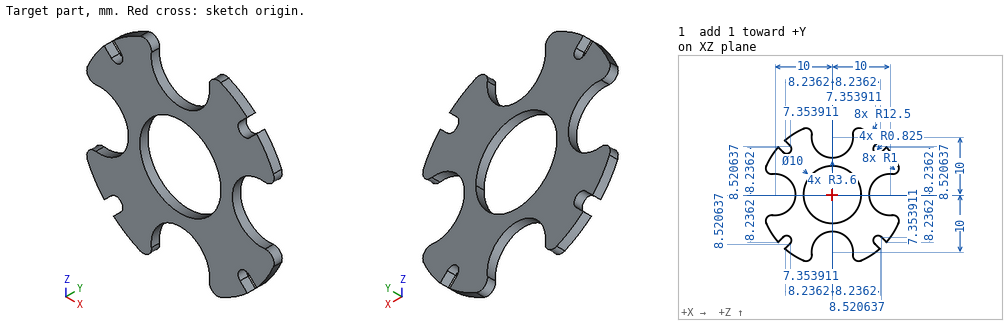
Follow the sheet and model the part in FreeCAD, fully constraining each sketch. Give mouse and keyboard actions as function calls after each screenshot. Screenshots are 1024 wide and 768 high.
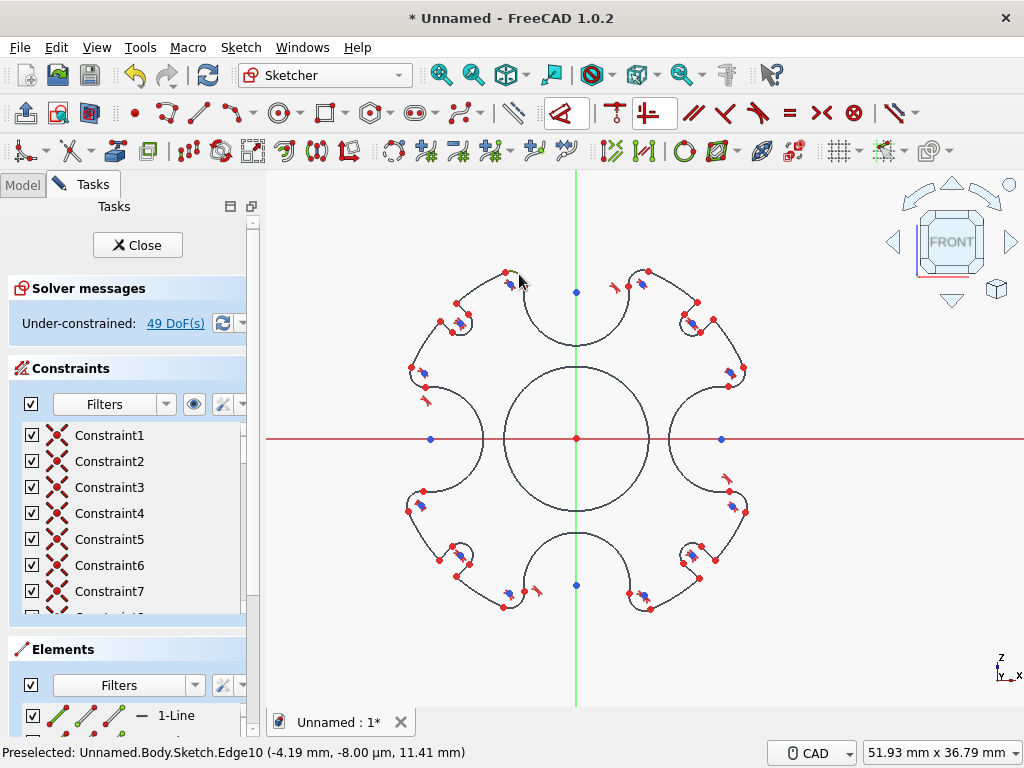
click(634, 273)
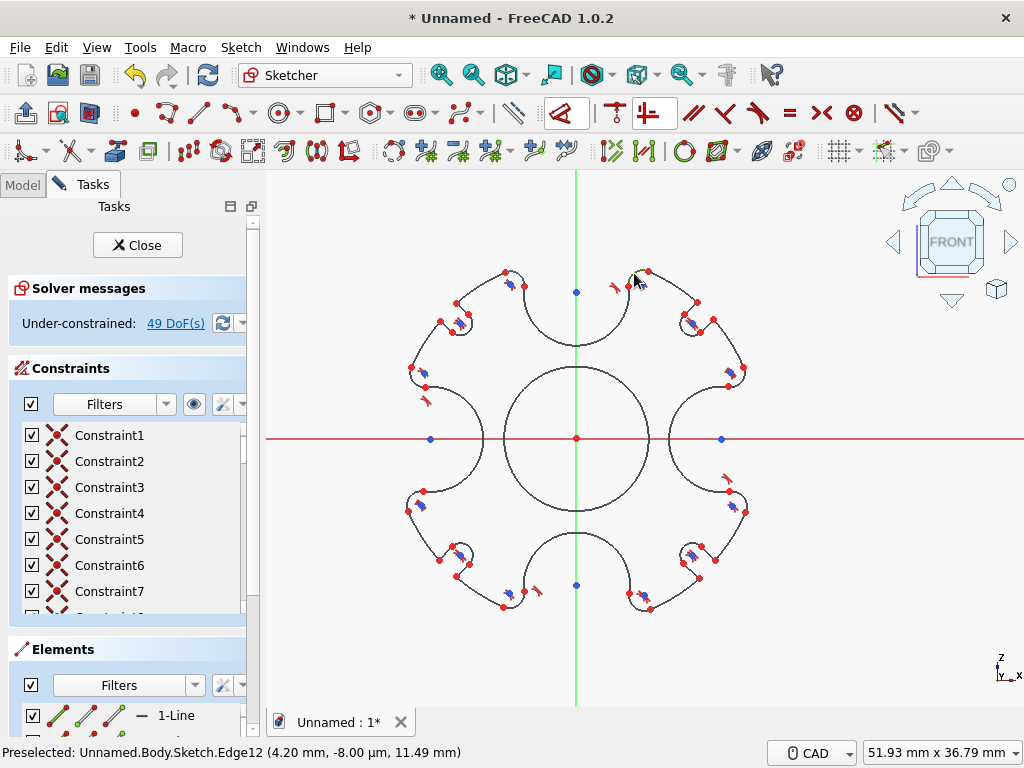
click(742, 381)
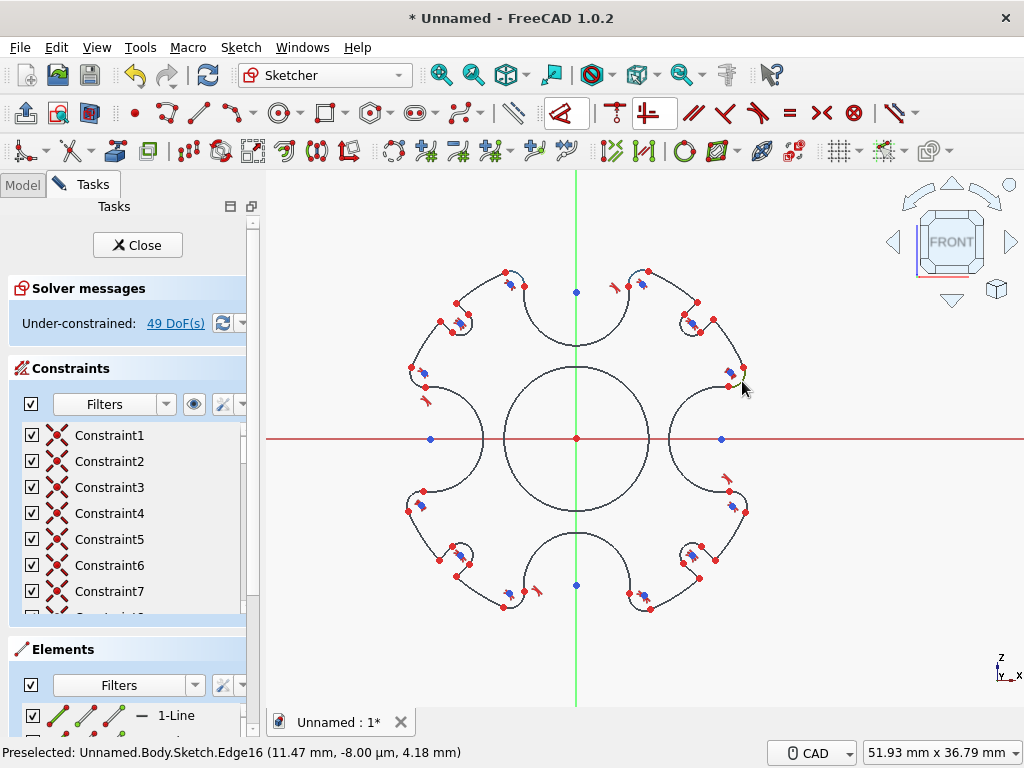
scroll(747, 503, up, 2)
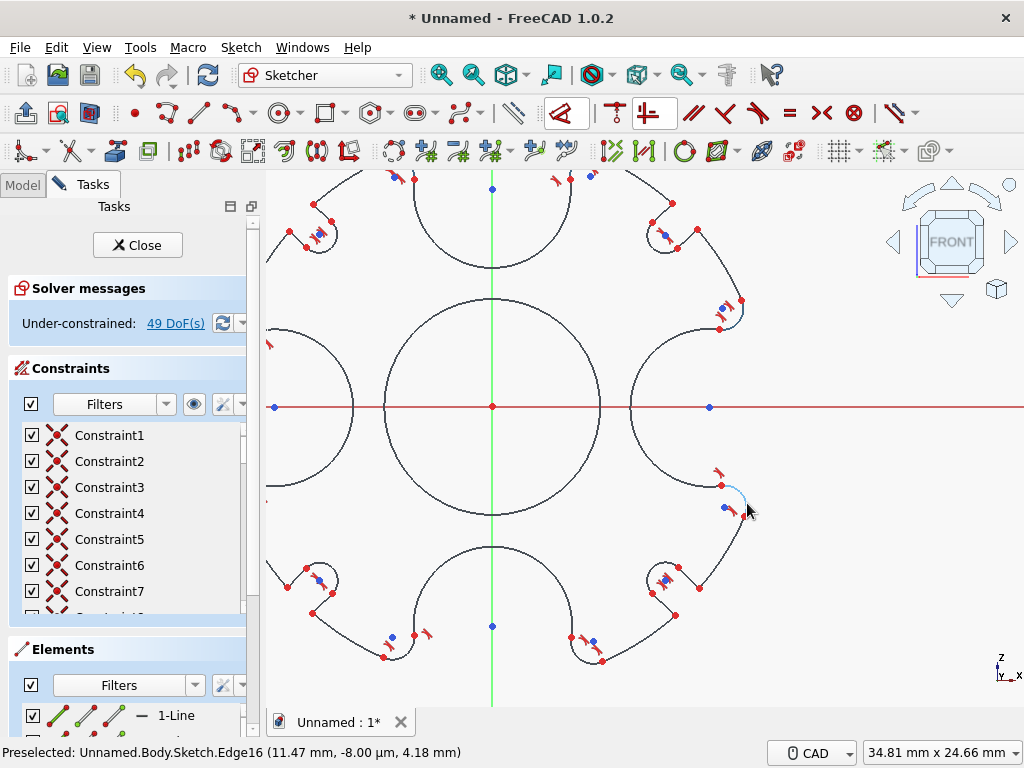
click(746, 503)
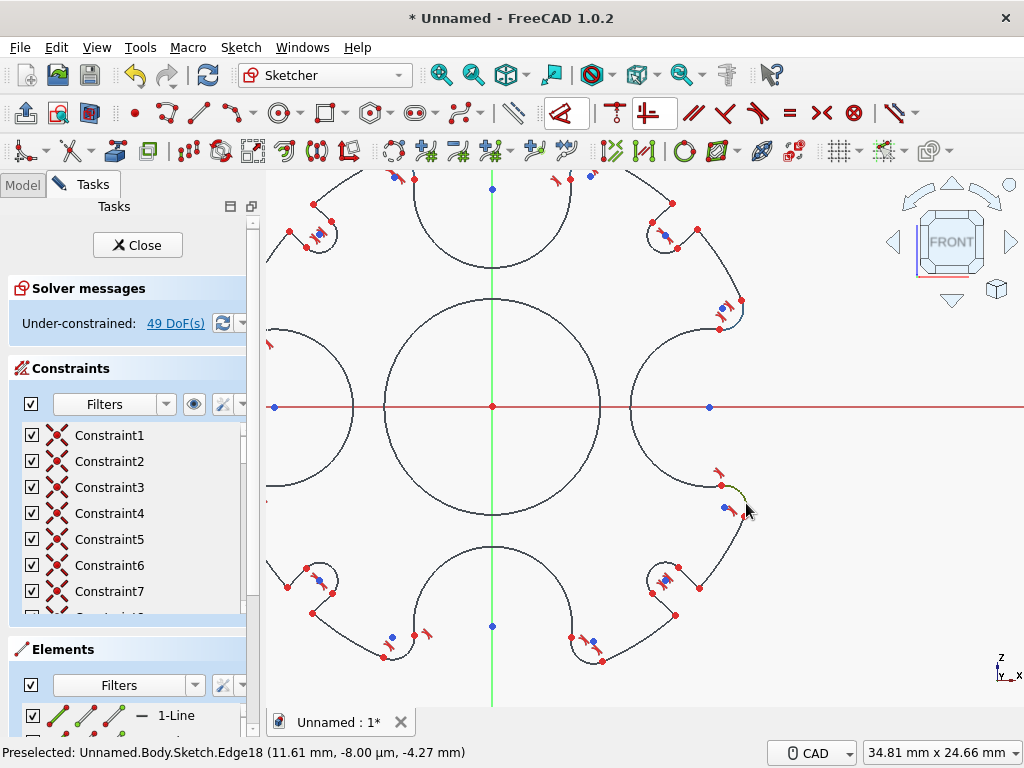
click(574, 652)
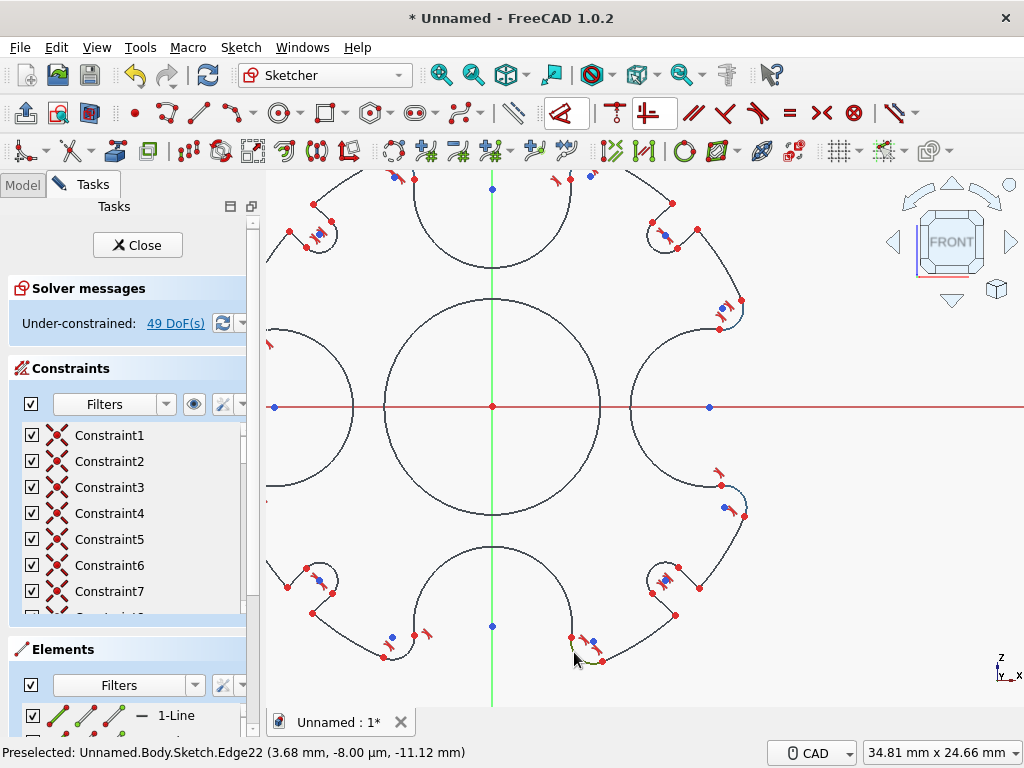
click(397, 659)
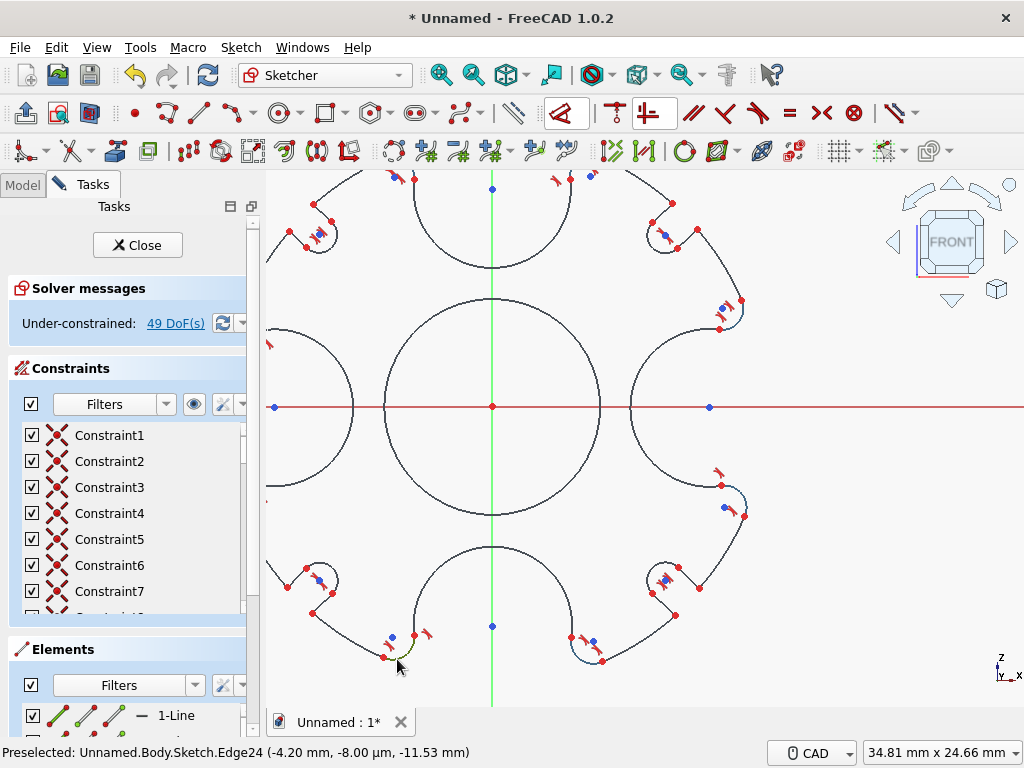
scroll(748, 503, down, 2)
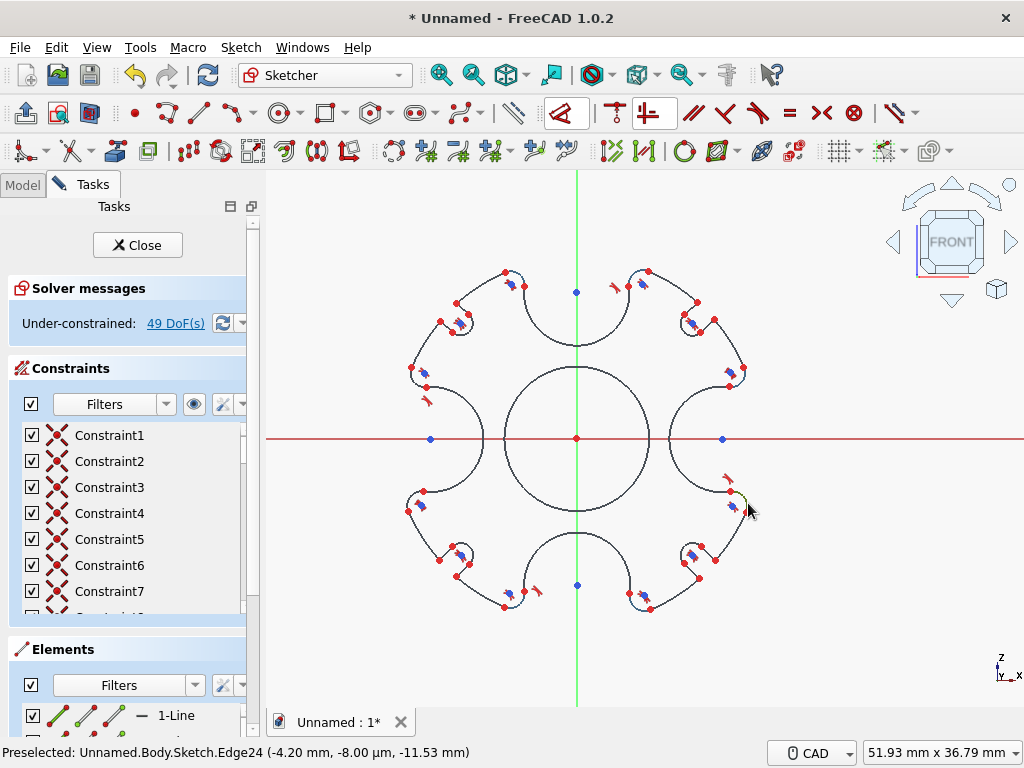
scroll(415, 493, up, 3)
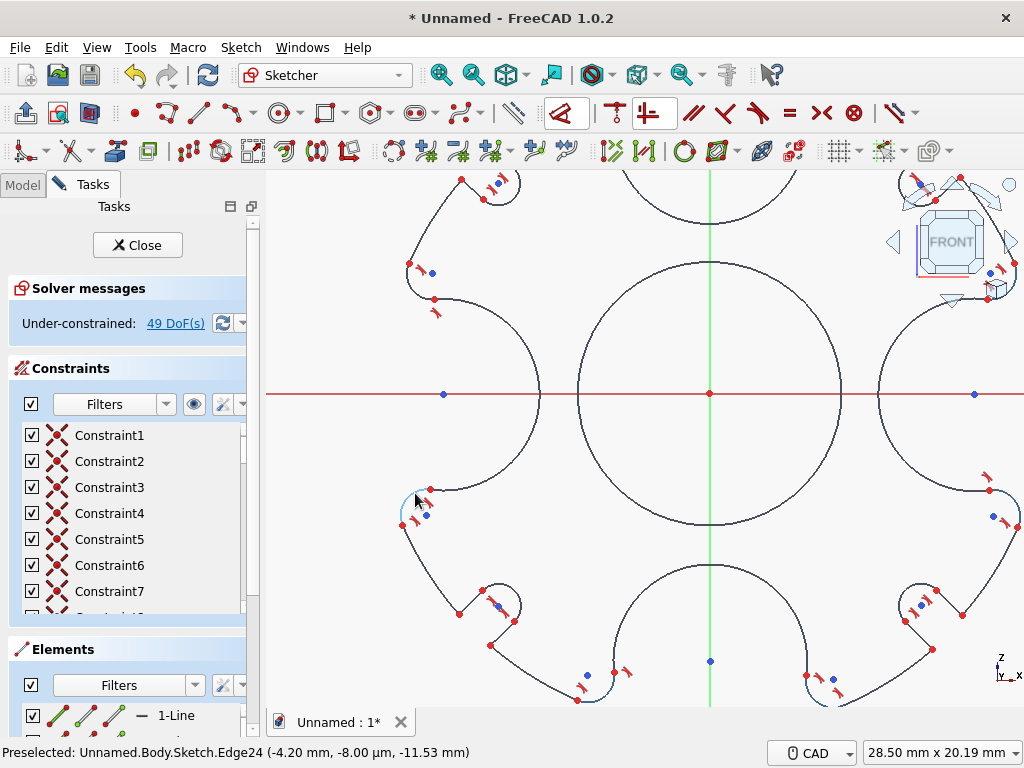
click(414, 492)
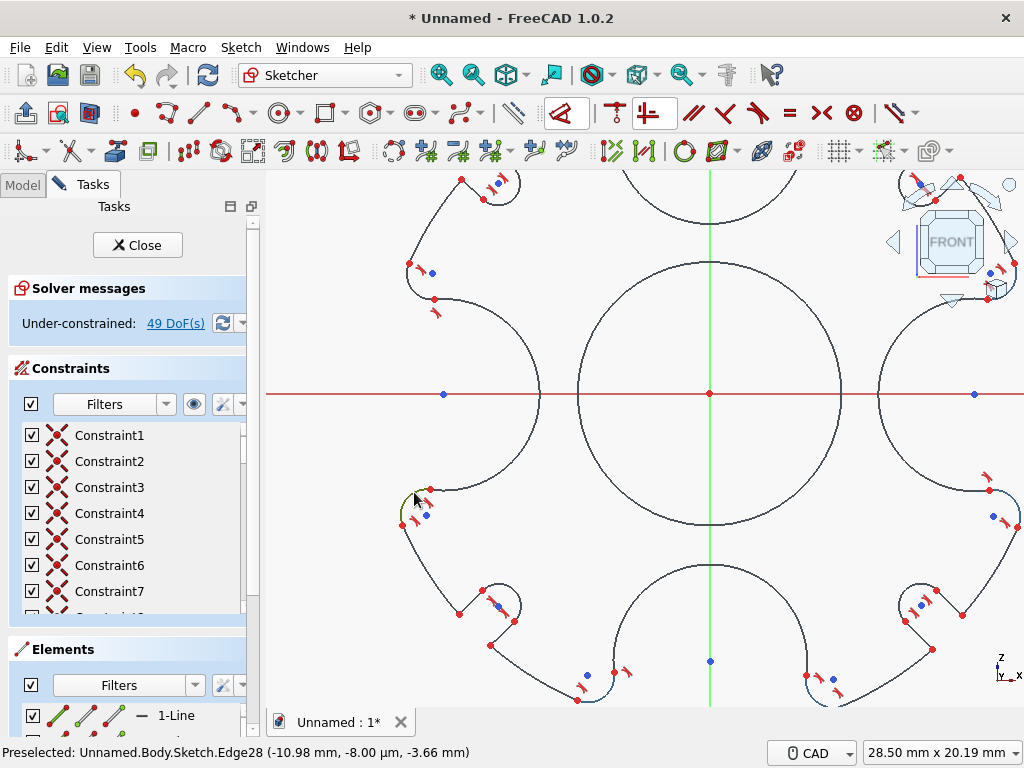
click(407, 279)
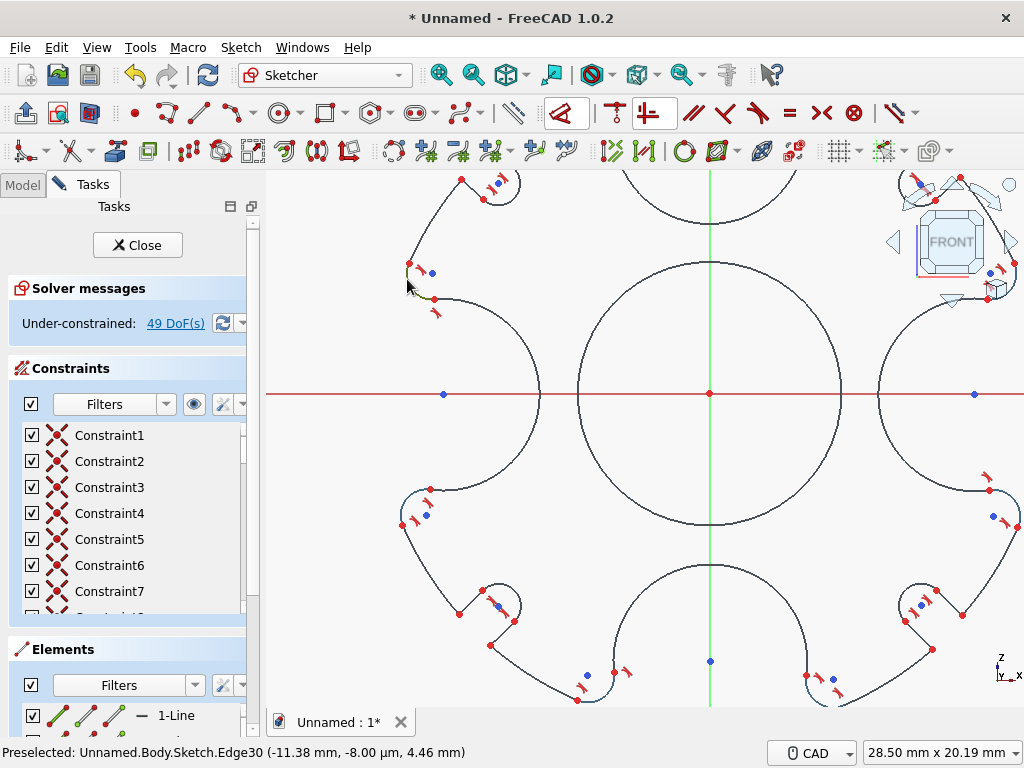
key(e)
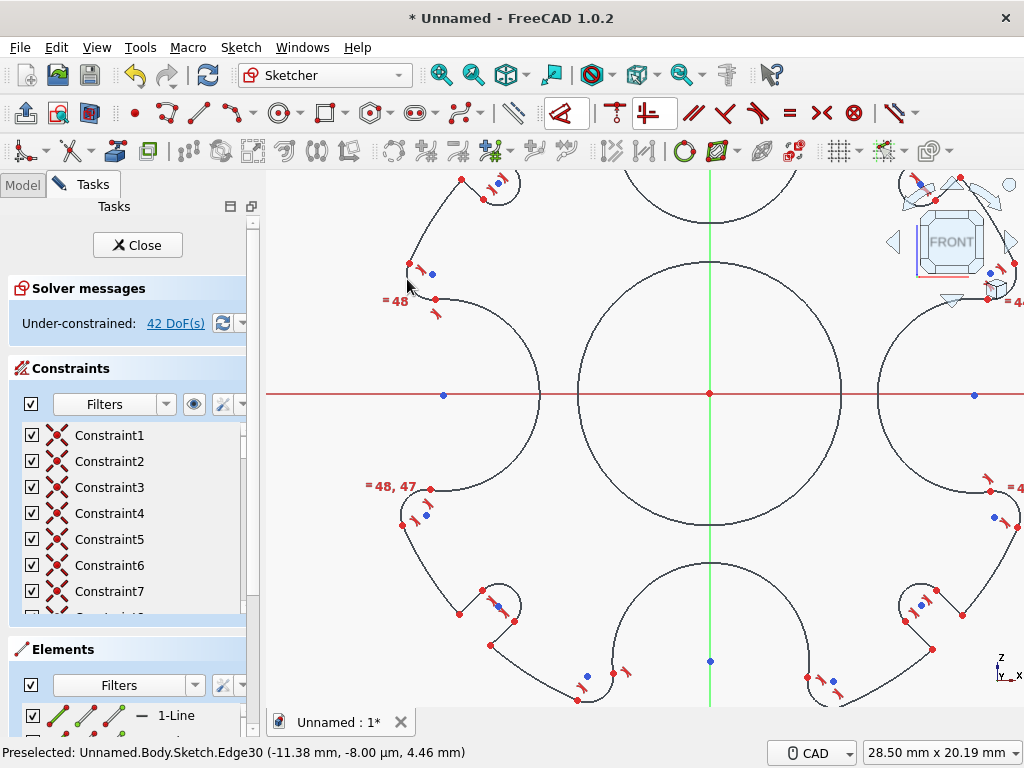
scroll(415, 493, down, 3)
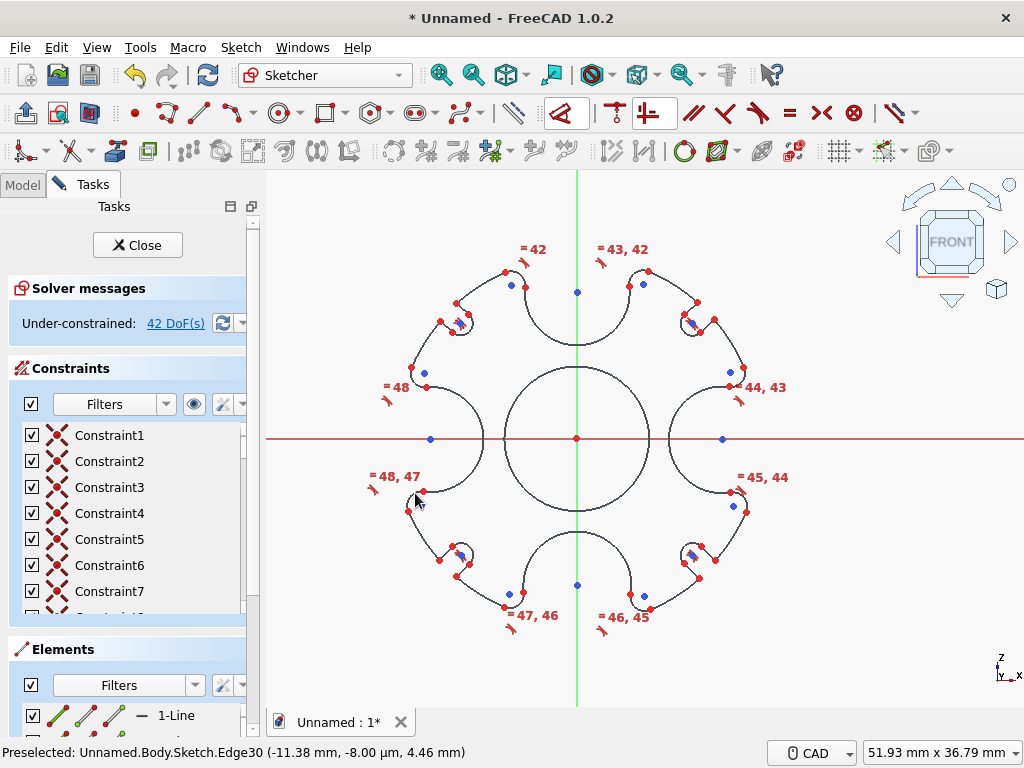
click(490, 280)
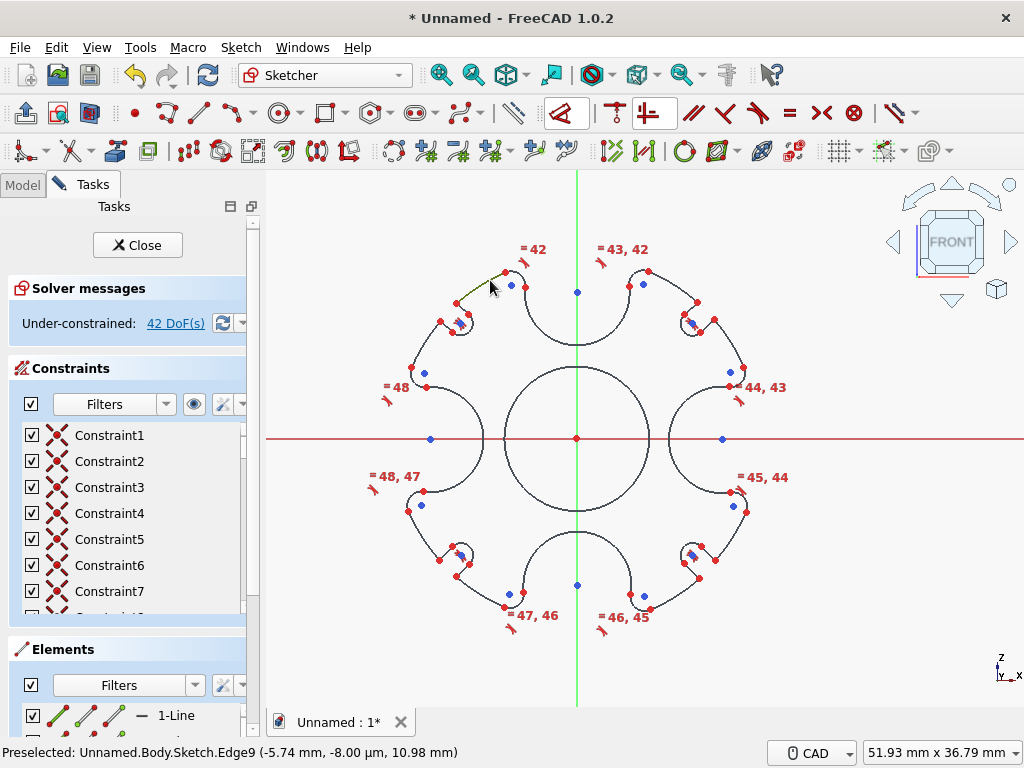
click(684, 292)